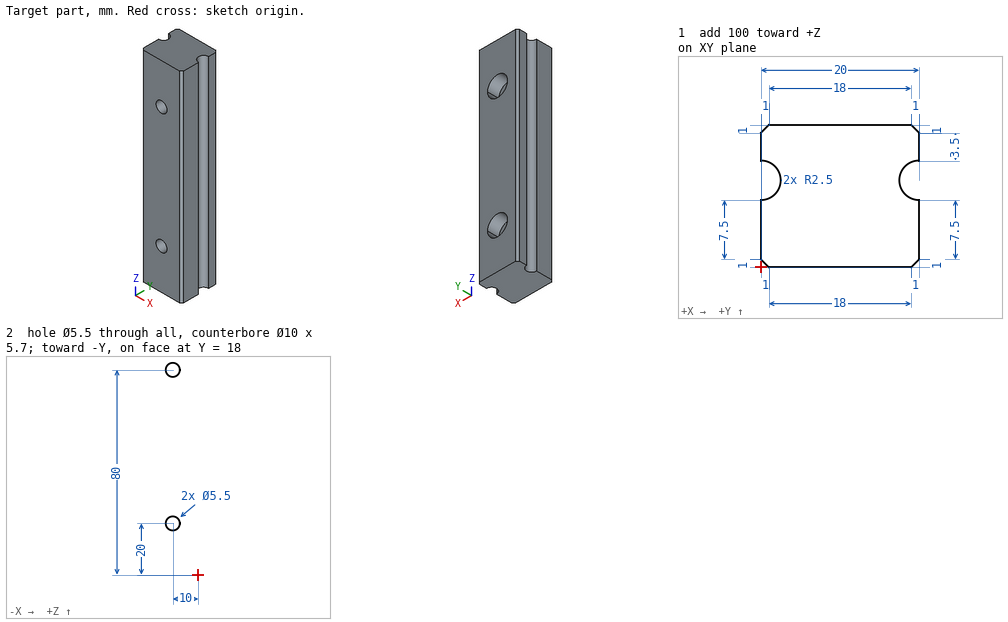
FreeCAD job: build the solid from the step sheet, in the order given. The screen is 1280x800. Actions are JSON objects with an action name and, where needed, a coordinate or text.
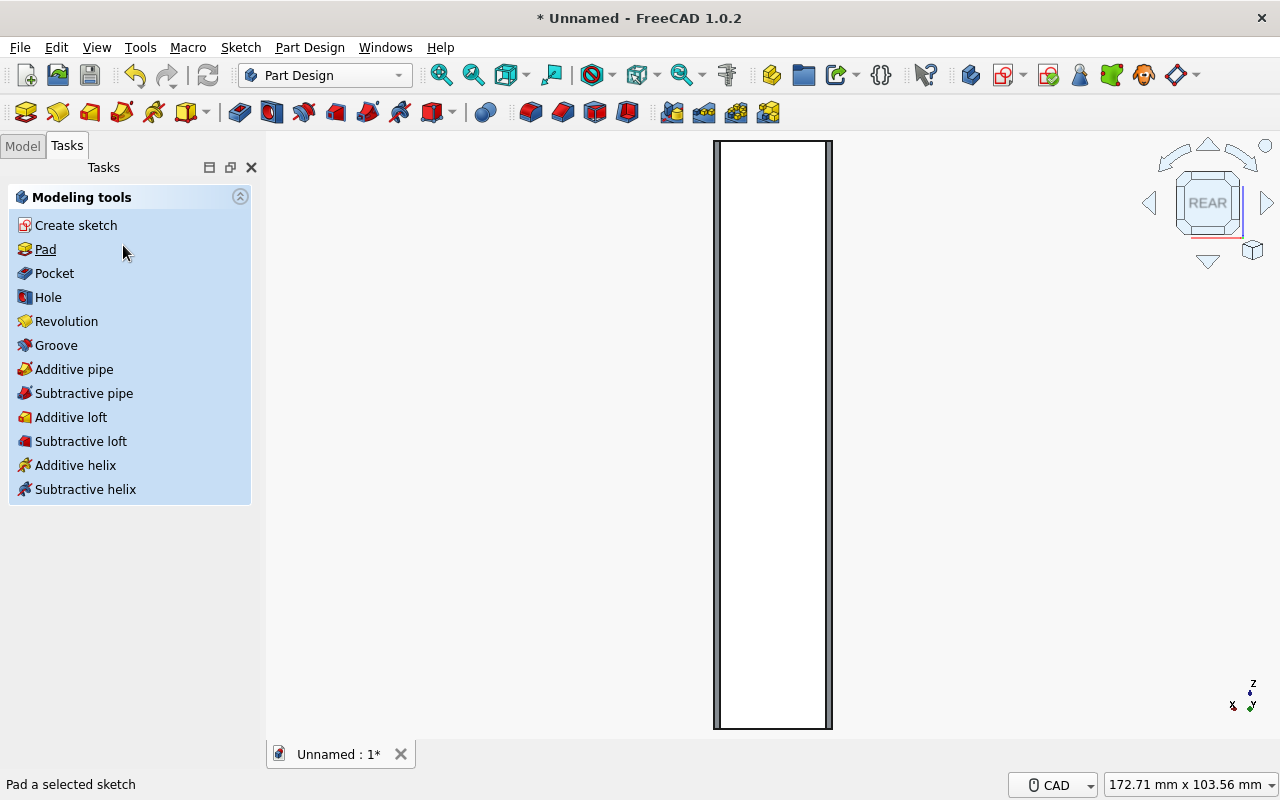
{"action": "left_click", "coordinate": [272, 112]}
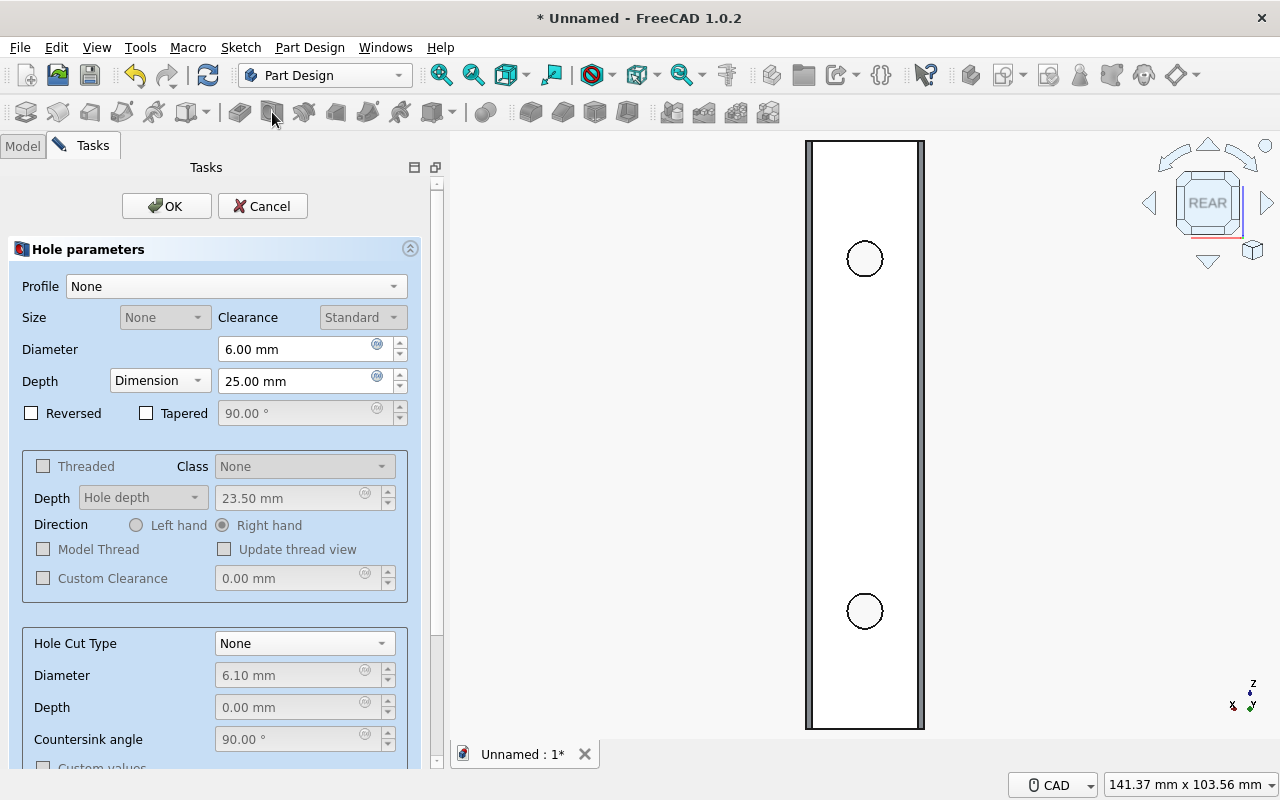
{"action": "triple_click", "coordinate": [305, 349]}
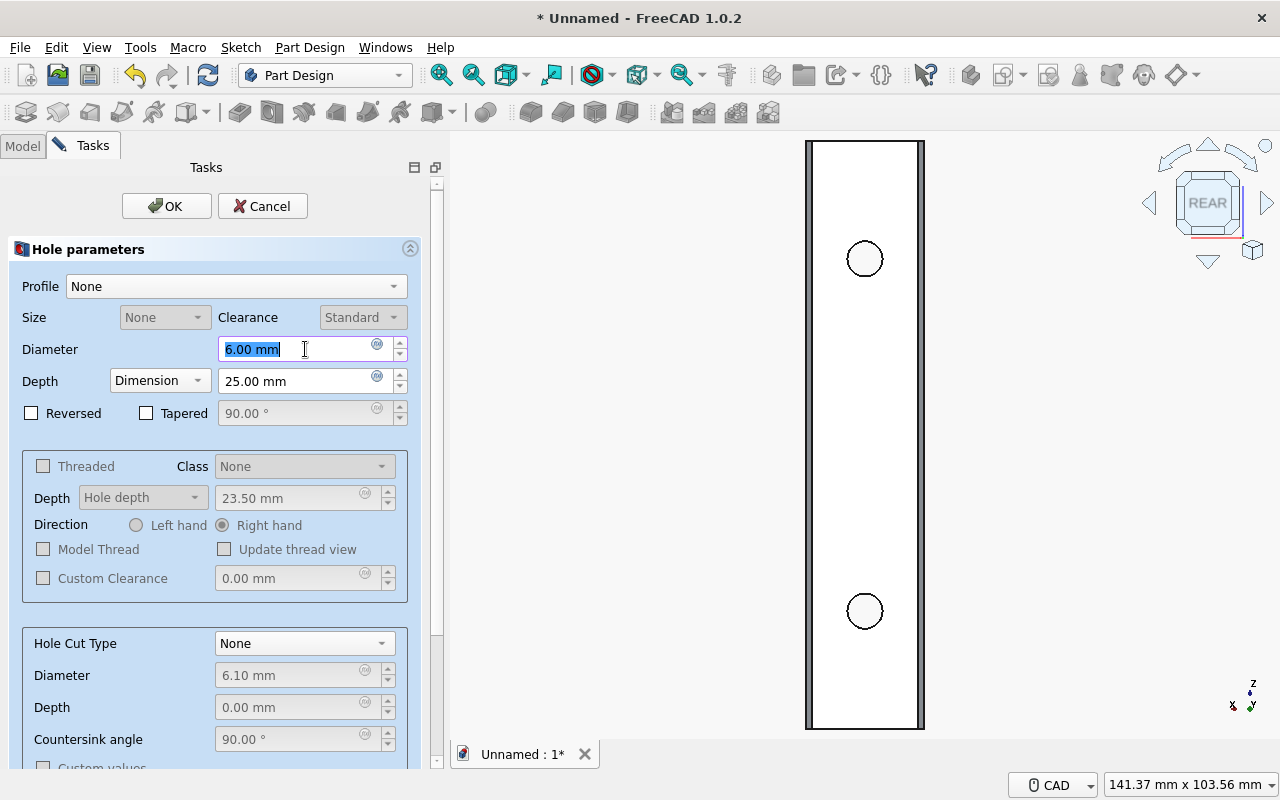
{"action": "type", "text": "5.5"}
{"action": "key", "text": "Tab"}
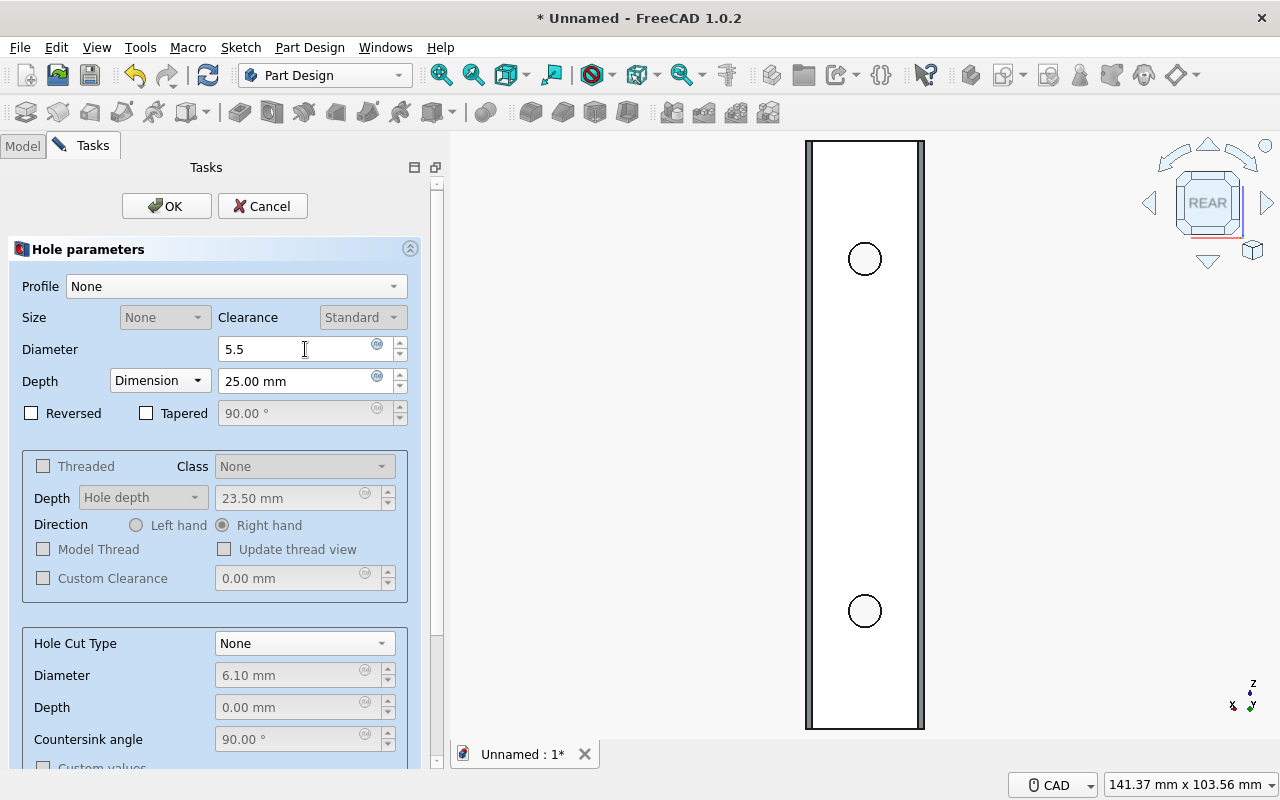
{"action": "left_click", "coordinate": [161, 380]}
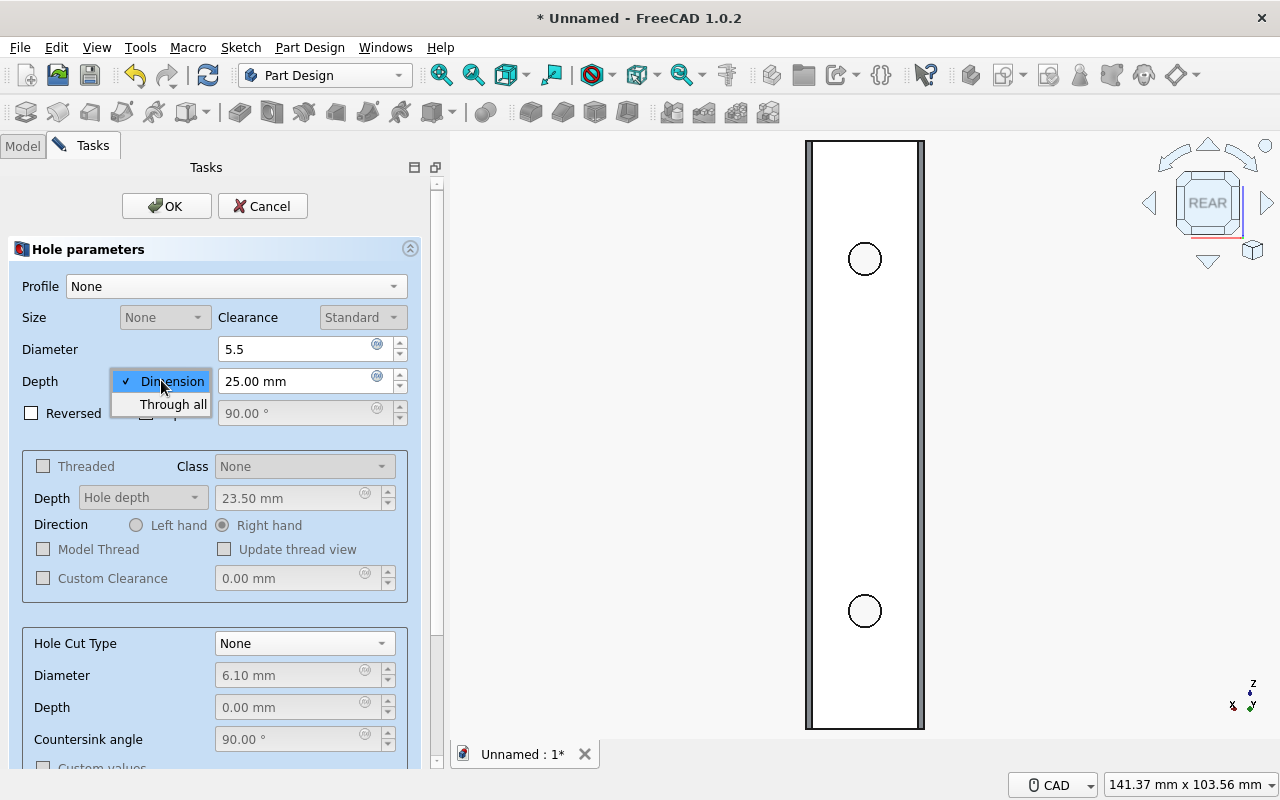
{"action": "left_click", "coordinate": [160, 404]}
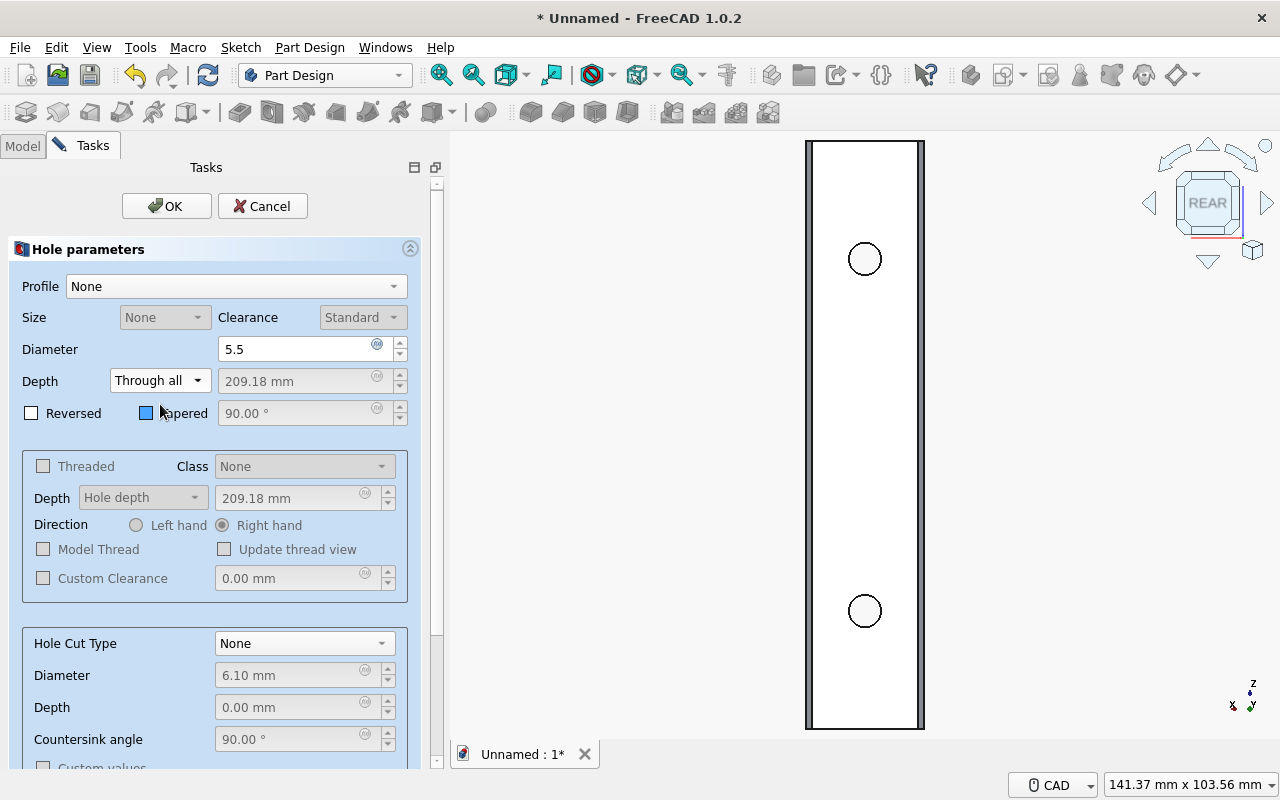
{"action": "left_click", "coordinate": [306, 644]}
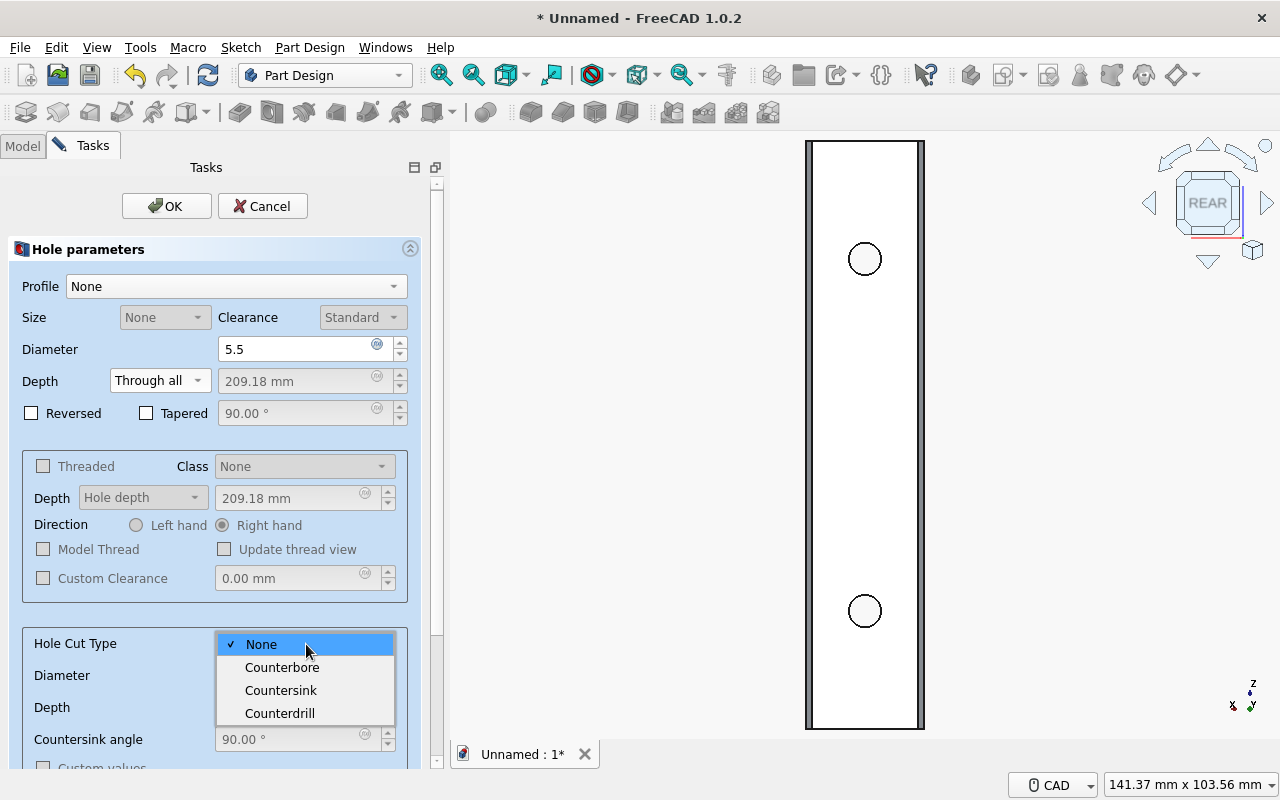
{"action": "left_click", "coordinate": [304, 668]}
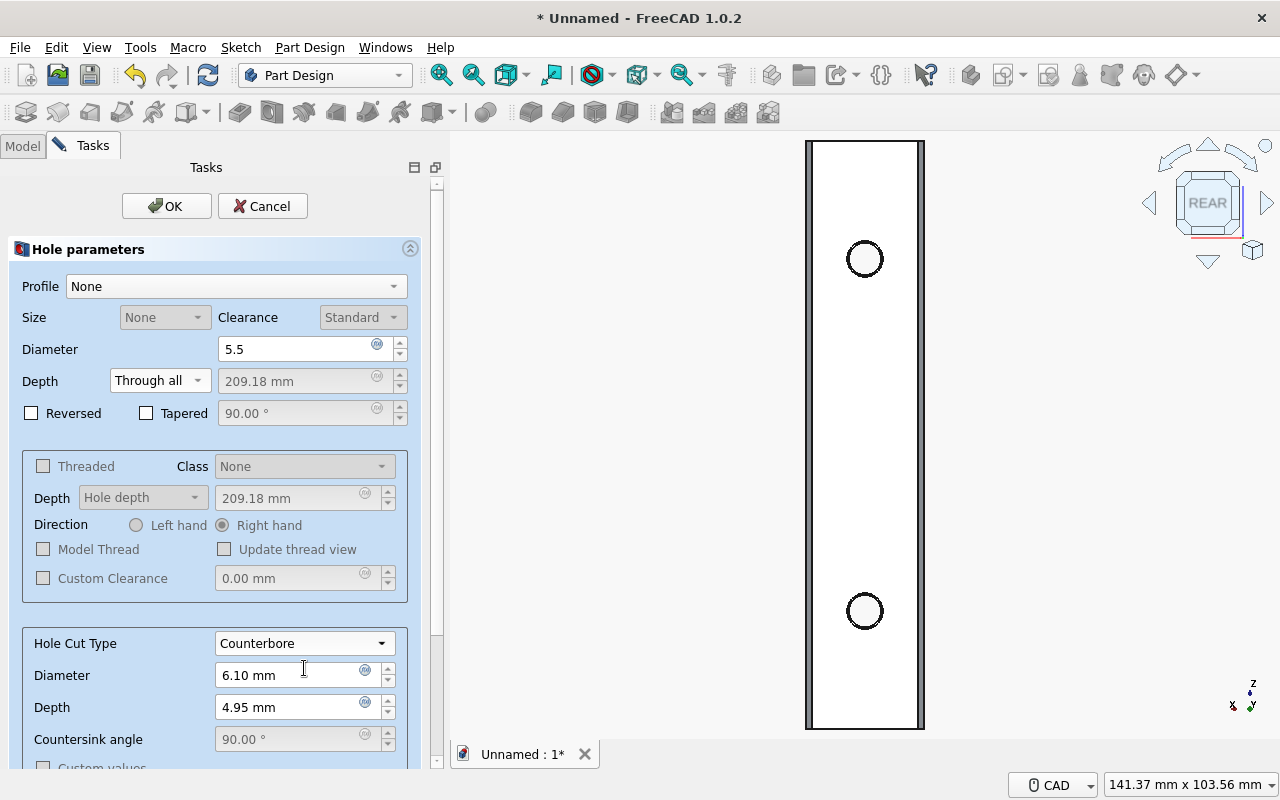
{"action": "triple_click", "coordinate": [298, 675]}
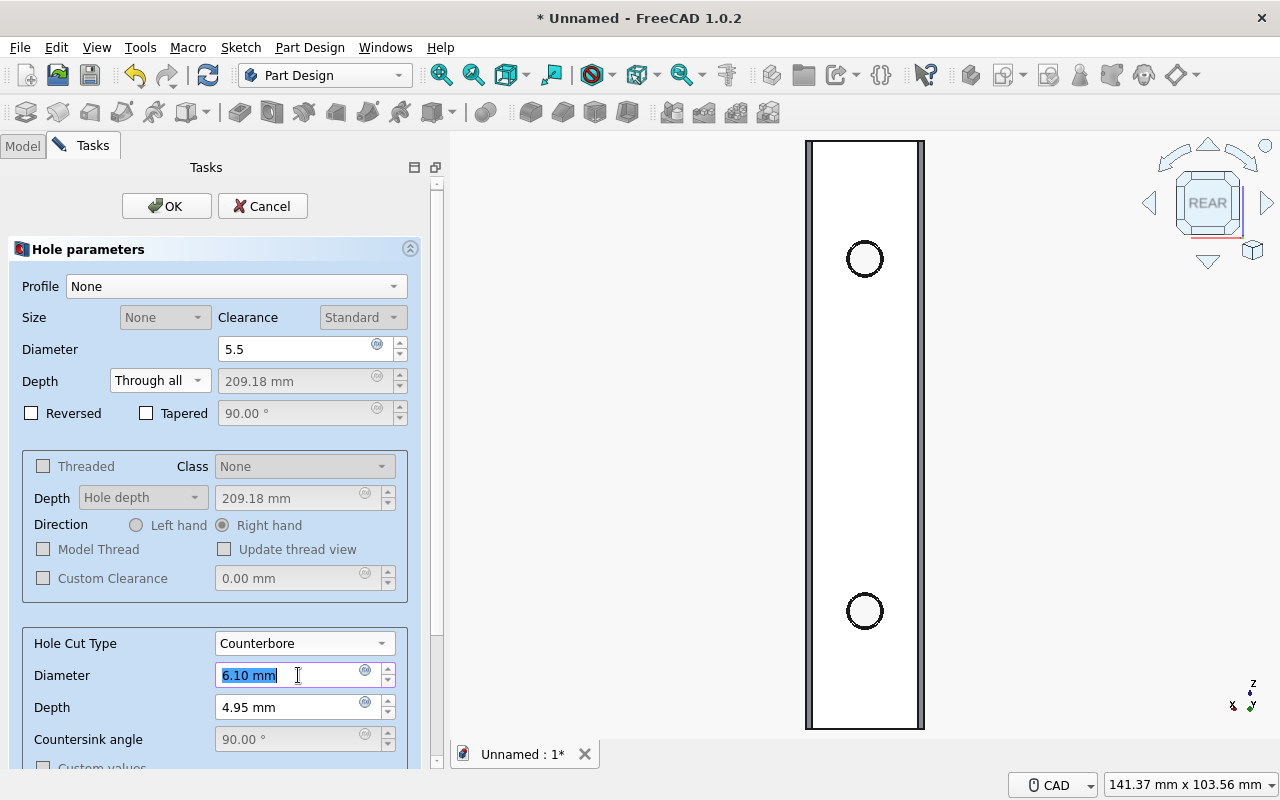
{"action": "type", "text": "10"}
{"action": "key", "text": "Tab"}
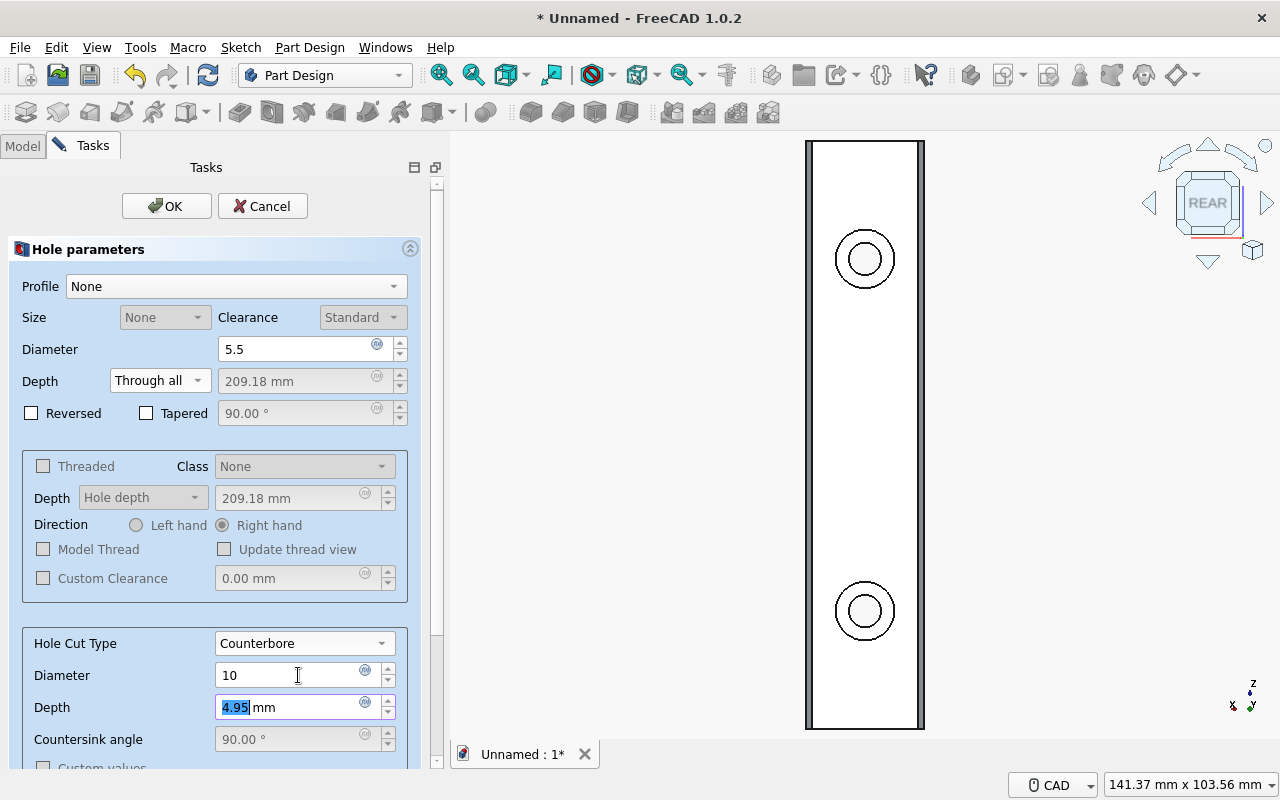
{"action": "type", "text": "5.7"}
{"action": "key", "text": "Tab"}